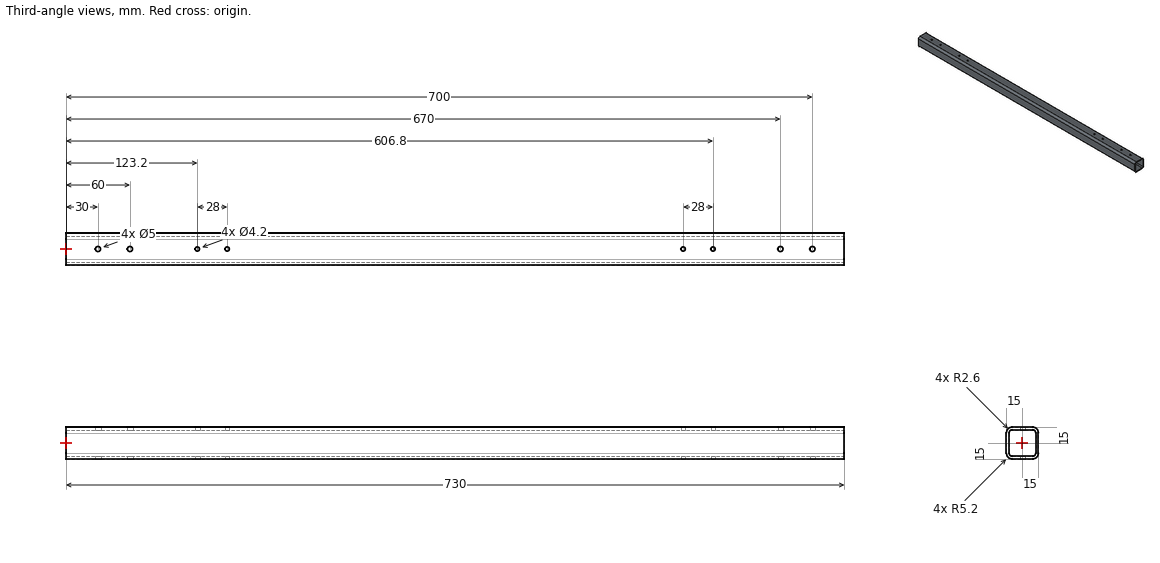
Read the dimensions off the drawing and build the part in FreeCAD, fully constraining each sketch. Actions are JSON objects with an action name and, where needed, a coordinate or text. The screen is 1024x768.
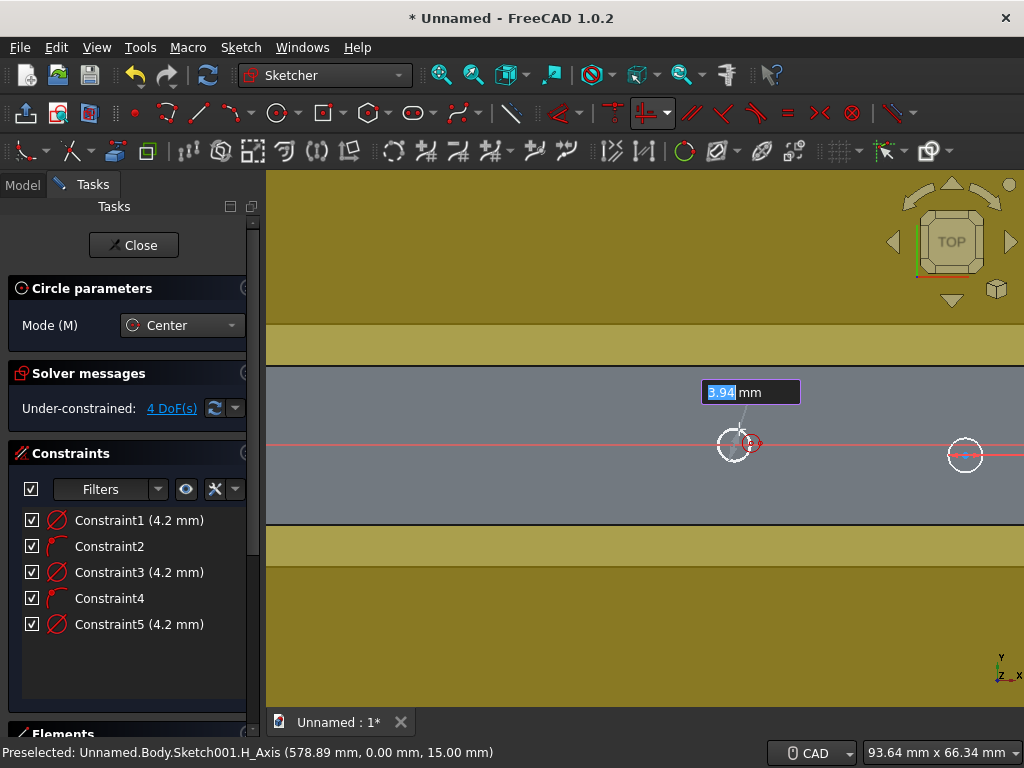
{"action": "type", "text": "4.2"}
{"action": "key", "text": "Return"}
{"action": "key", "text": "Escape"}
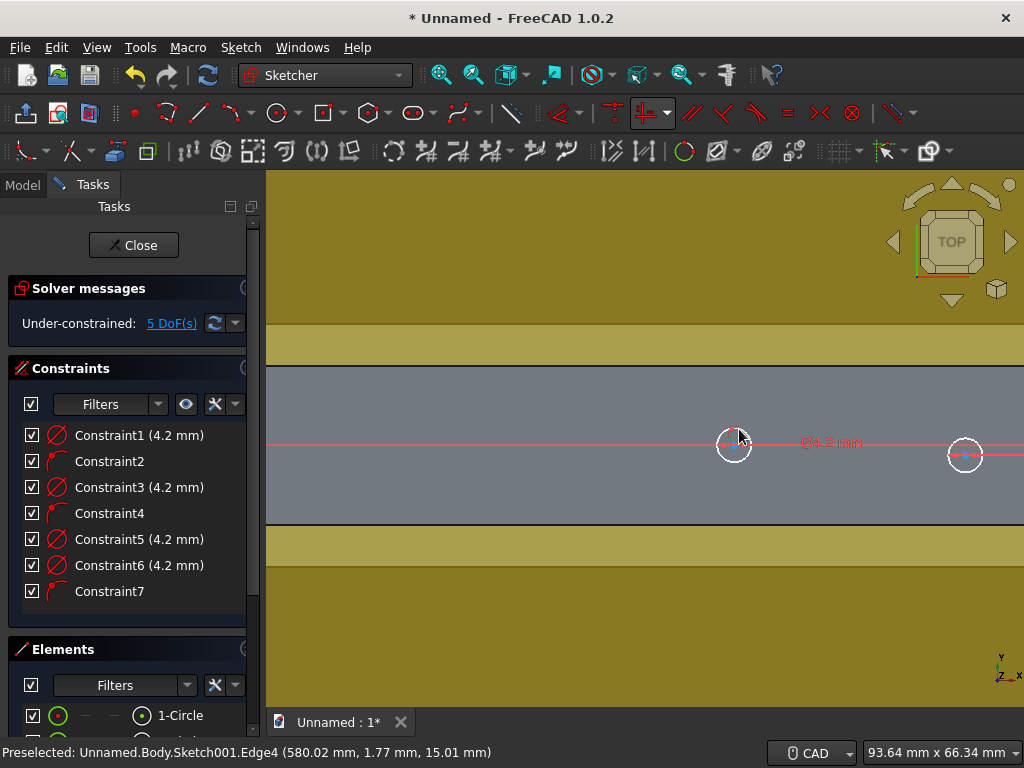
{"action": "scroll", "coordinate": [742, 438], "scroll_direction": "down", "scroll_amount": 13}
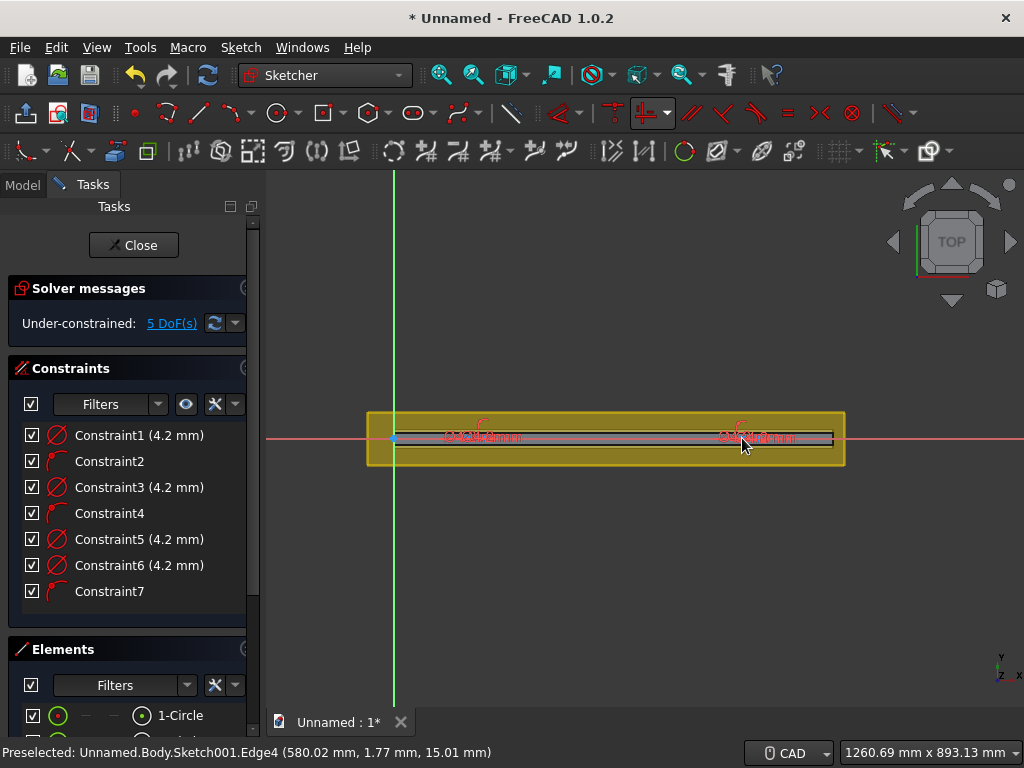
{"action": "left_click", "coordinate": [759, 440]}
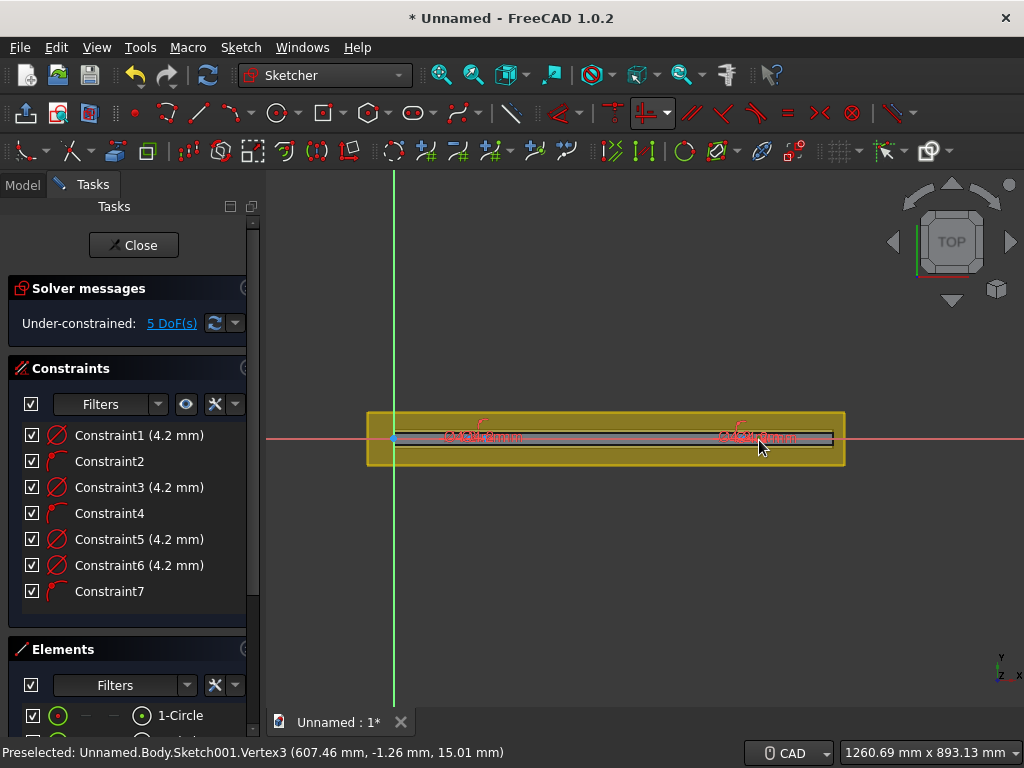
{"action": "left_click", "coordinate": [334, 439]}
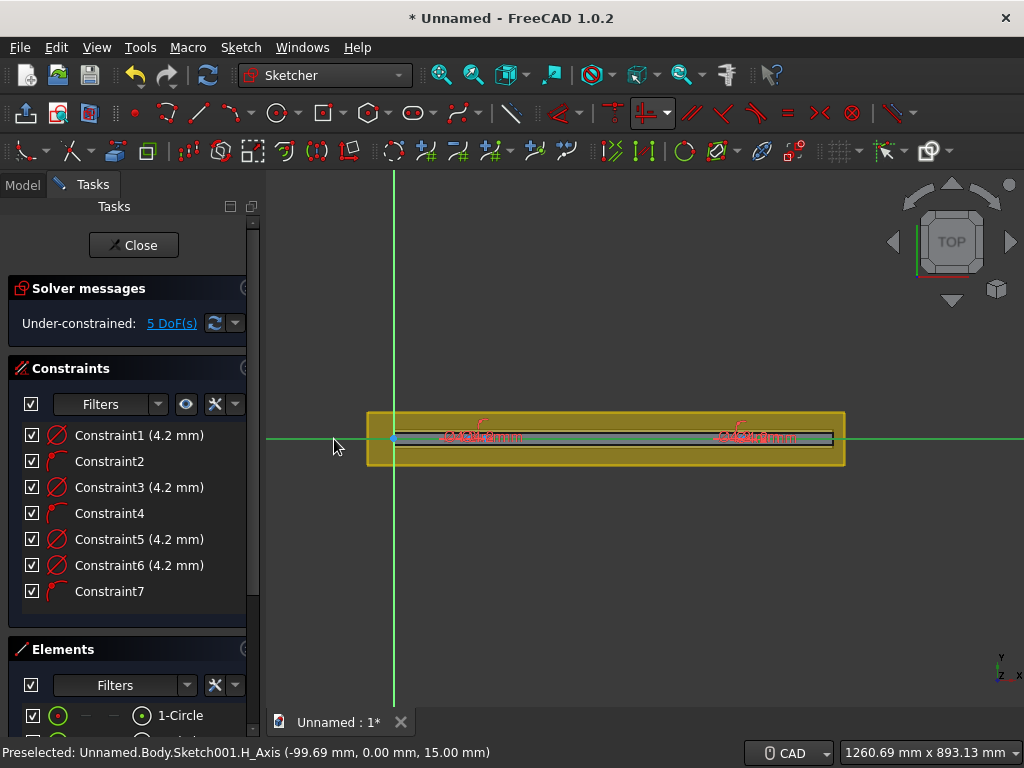
{"action": "left_click", "coordinate": [614, 114]}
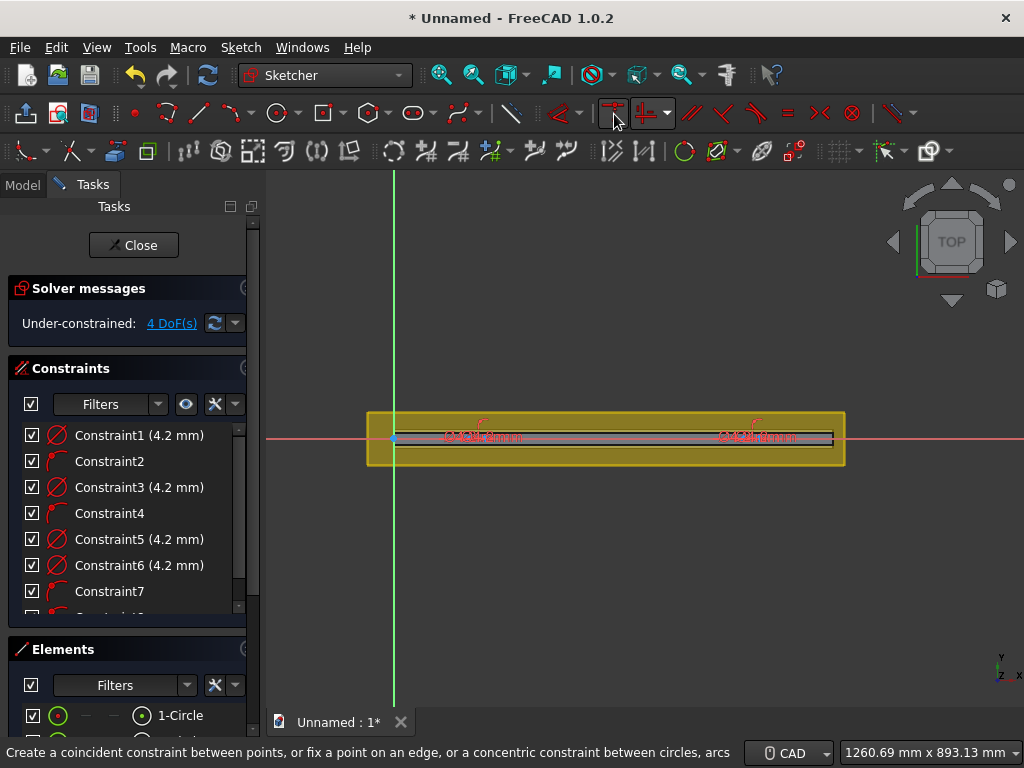
{"action": "left_click", "coordinate": [558, 114]}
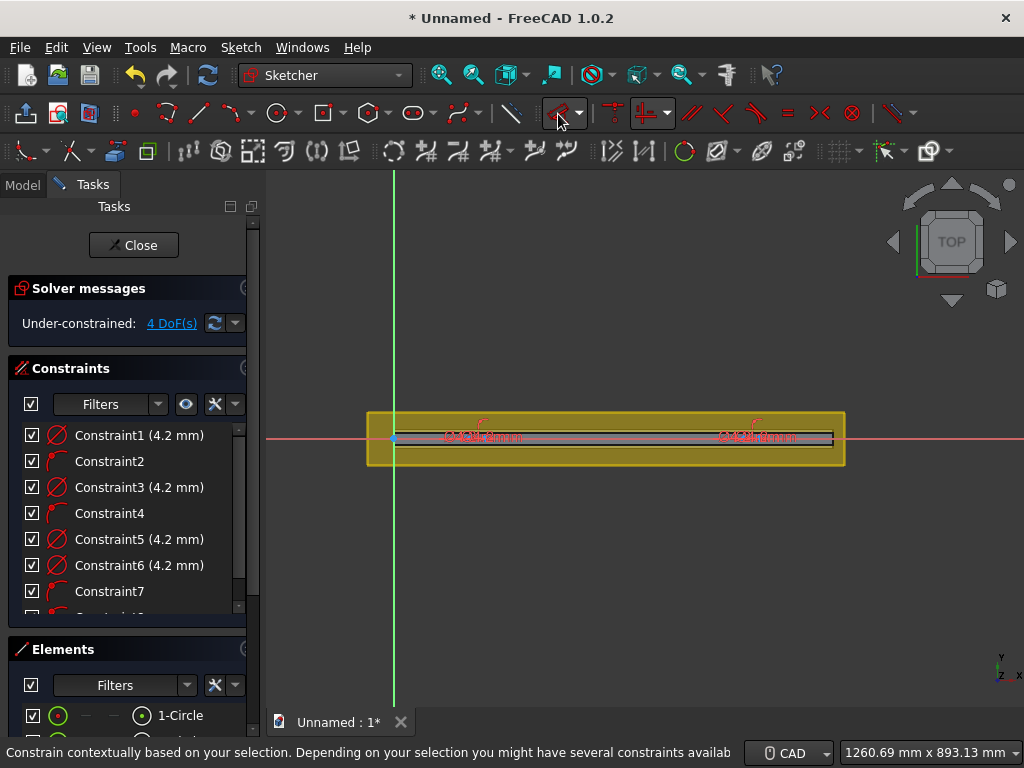
{"action": "scroll", "coordinate": [468, 439], "scroll_direction": "up", "scroll_amount": 5}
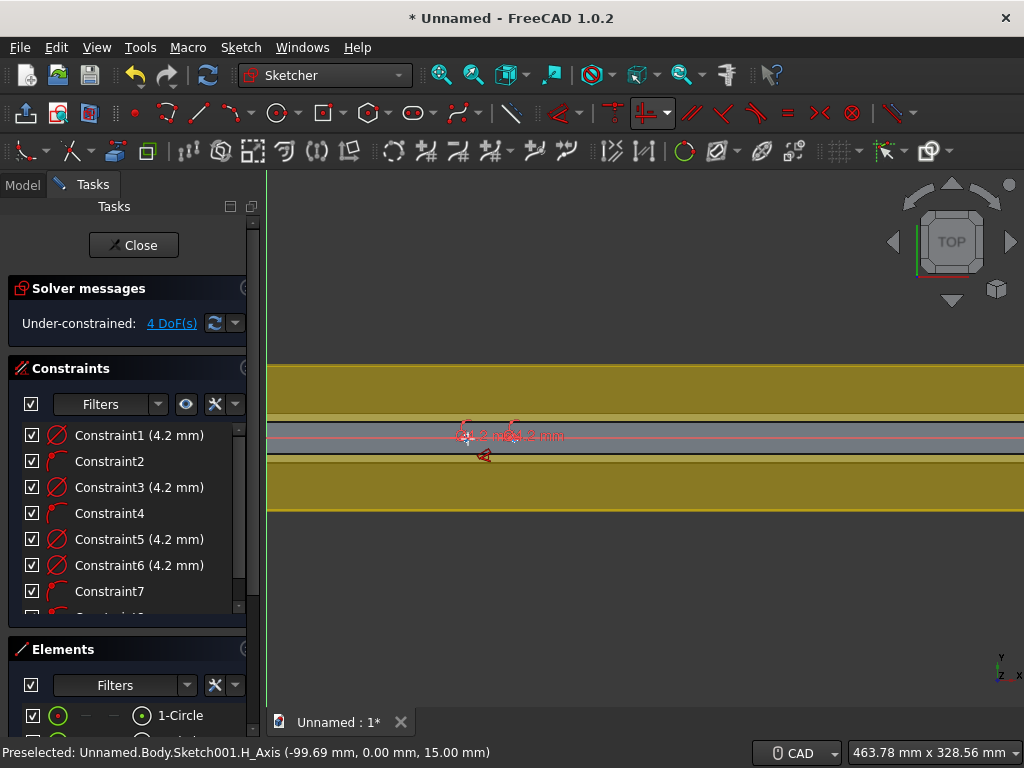
{"action": "left_click", "coordinate": [466, 438]}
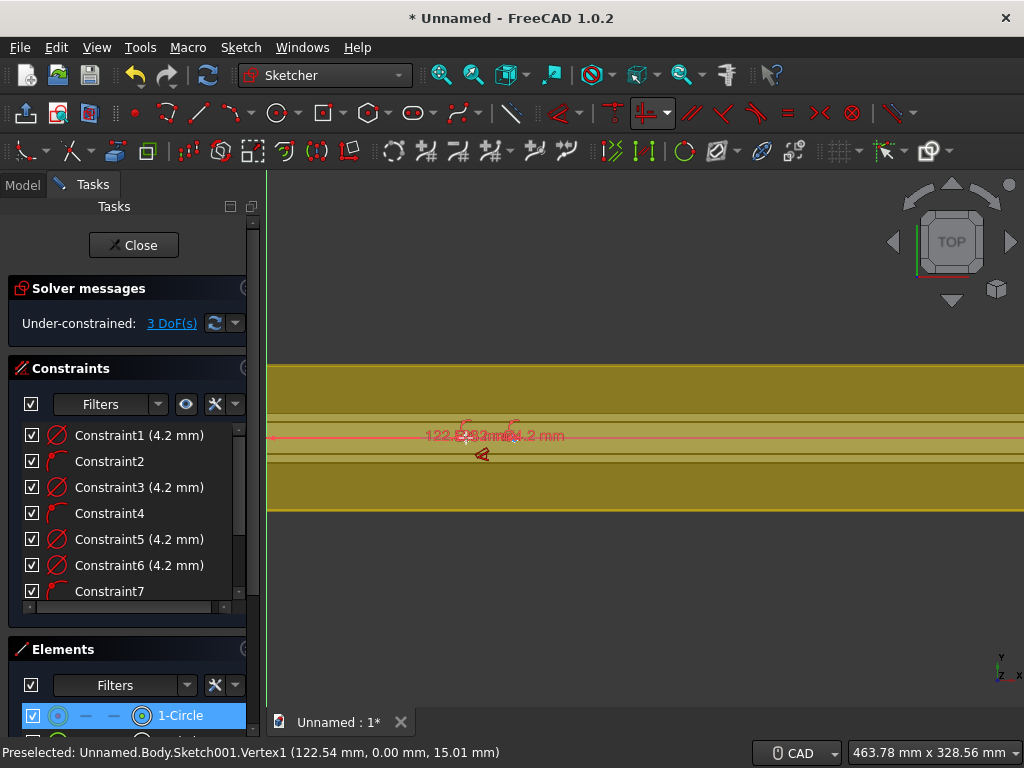
{"action": "left_click", "coordinate": [514, 438]}
{"action": "left_click", "coordinate": [490, 472]}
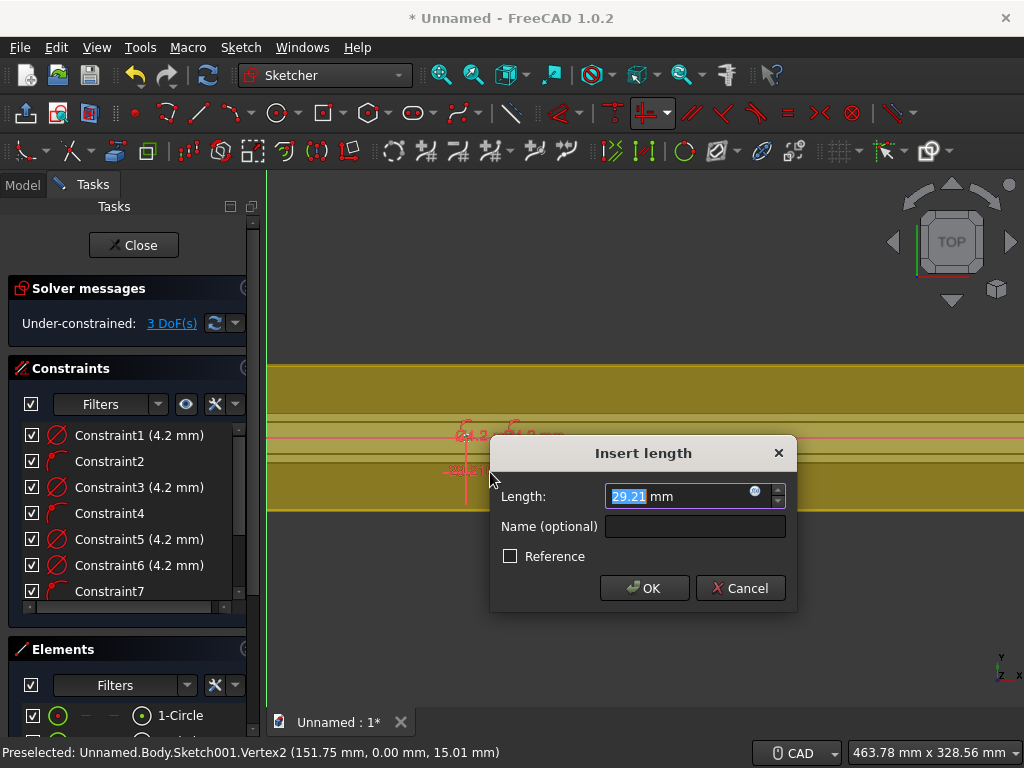
{"action": "type", "text": "28"}
{"action": "key", "text": "Return"}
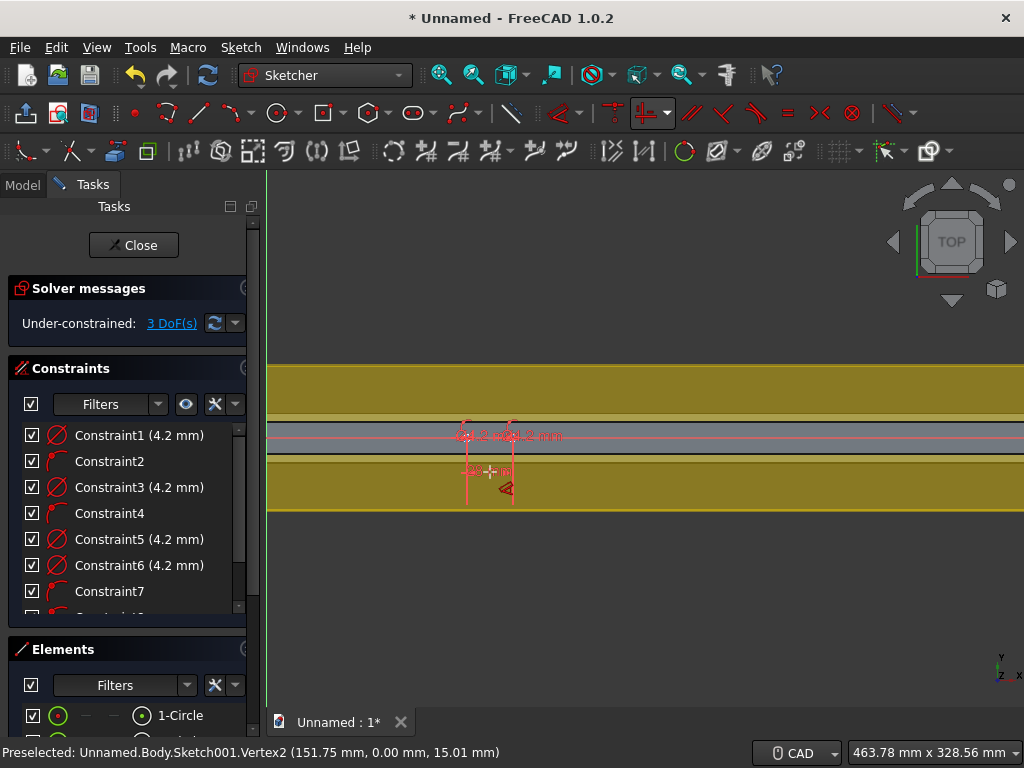
{"action": "scroll", "coordinate": [467, 439], "scroll_direction": "down", "scroll_amount": 5}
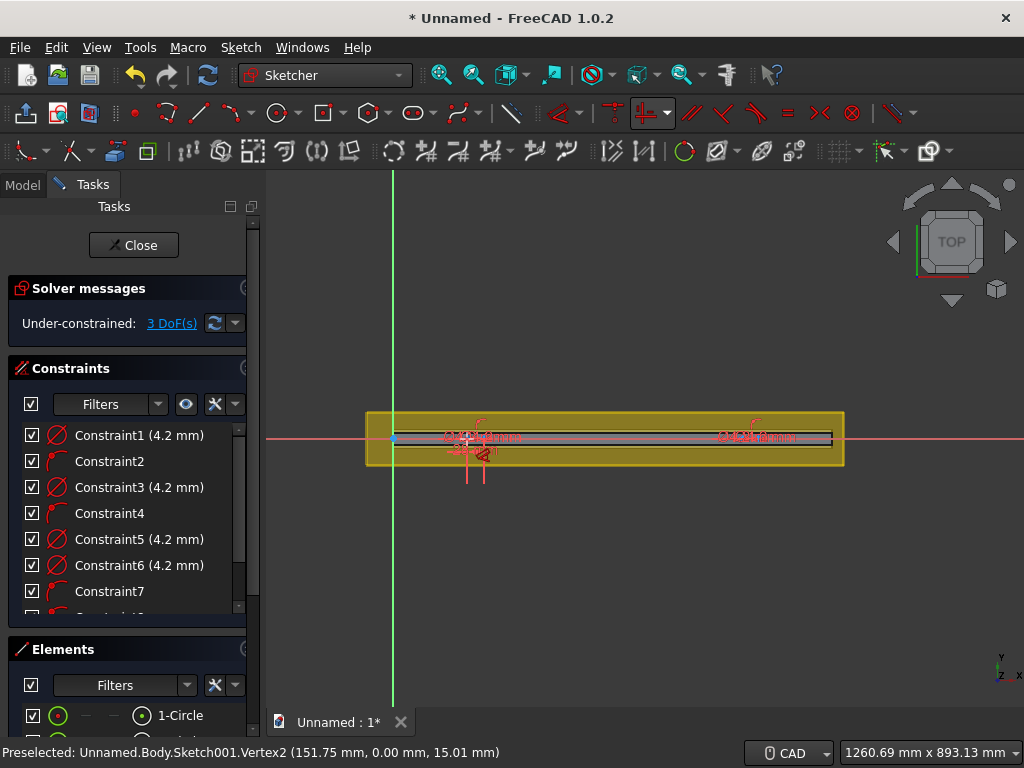
{"action": "scroll", "coordinate": [759, 439], "scroll_direction": "up", "scroll_amount": 5}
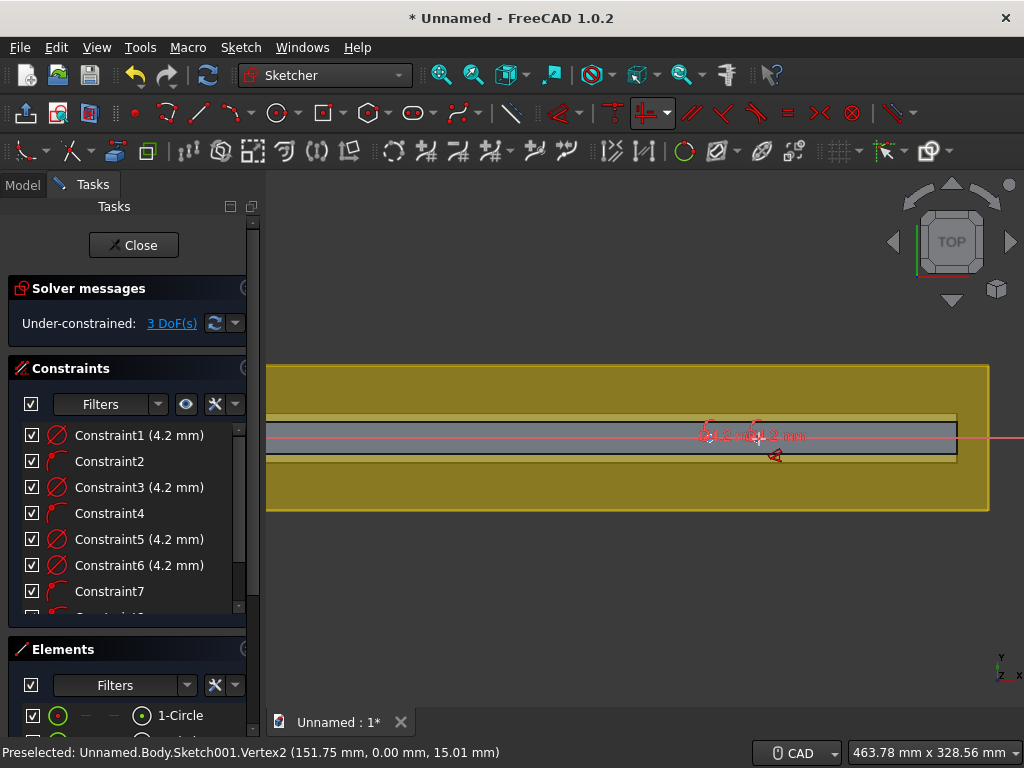
{"action": "left_click", "coordinate": [757, 438]}